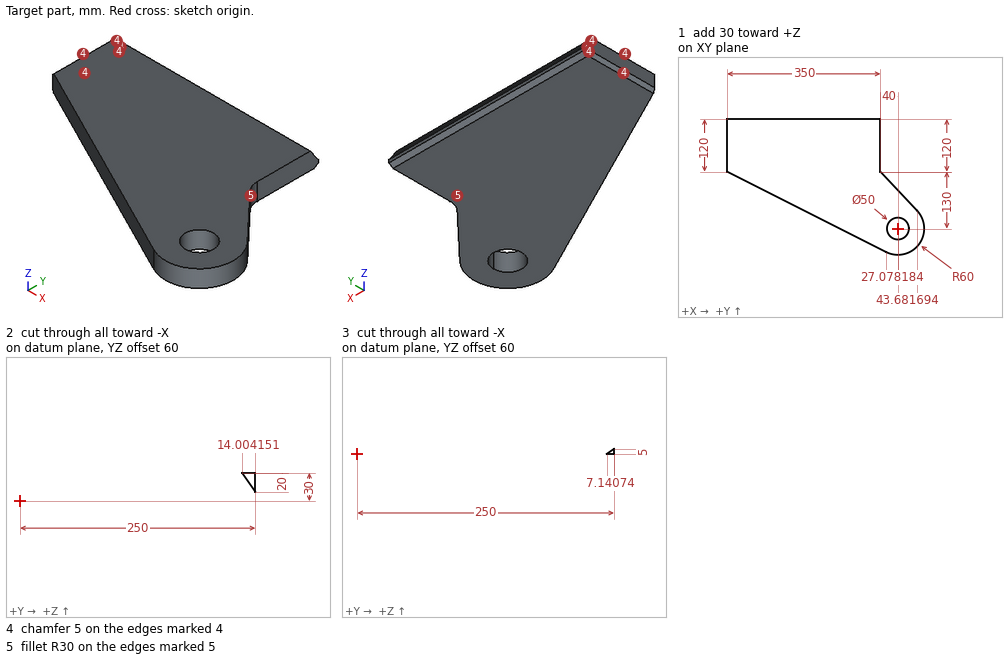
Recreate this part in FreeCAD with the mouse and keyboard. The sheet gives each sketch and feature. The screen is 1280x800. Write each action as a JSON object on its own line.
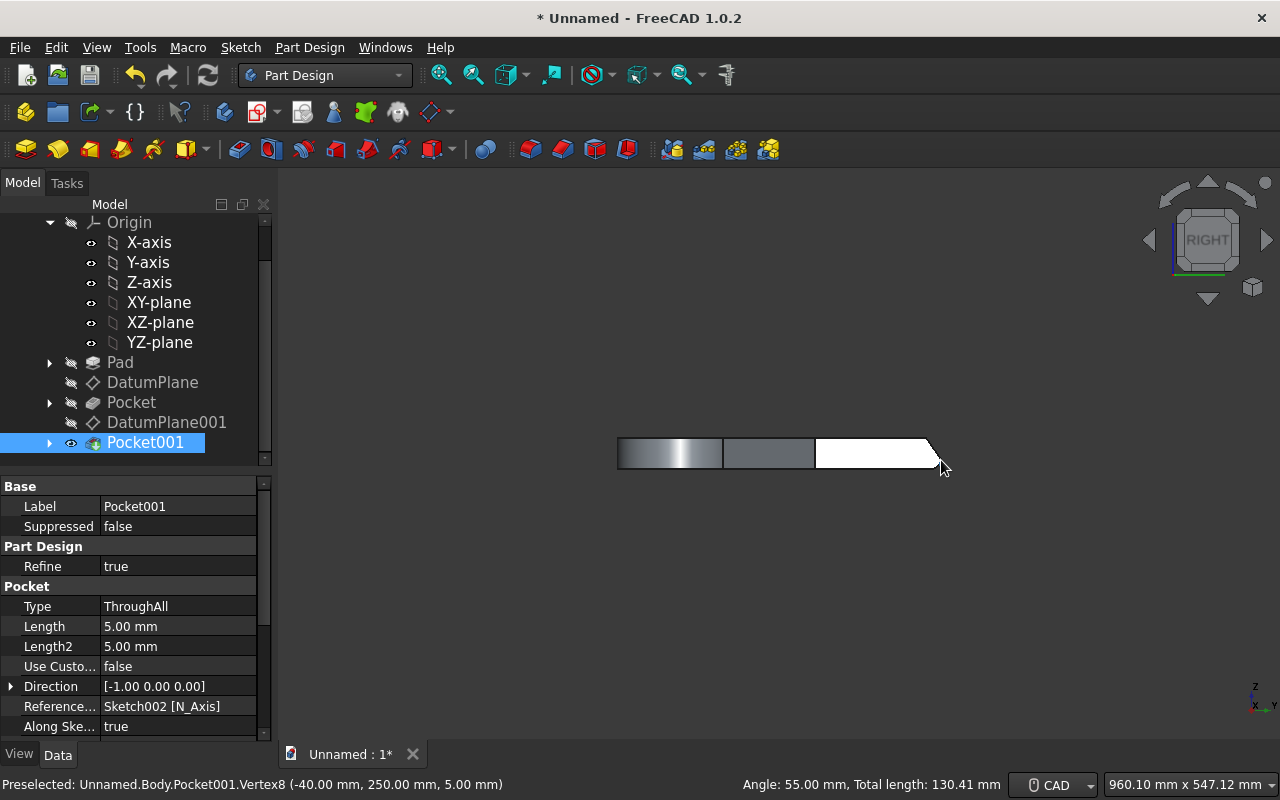
{"action": "key", "text": "5"}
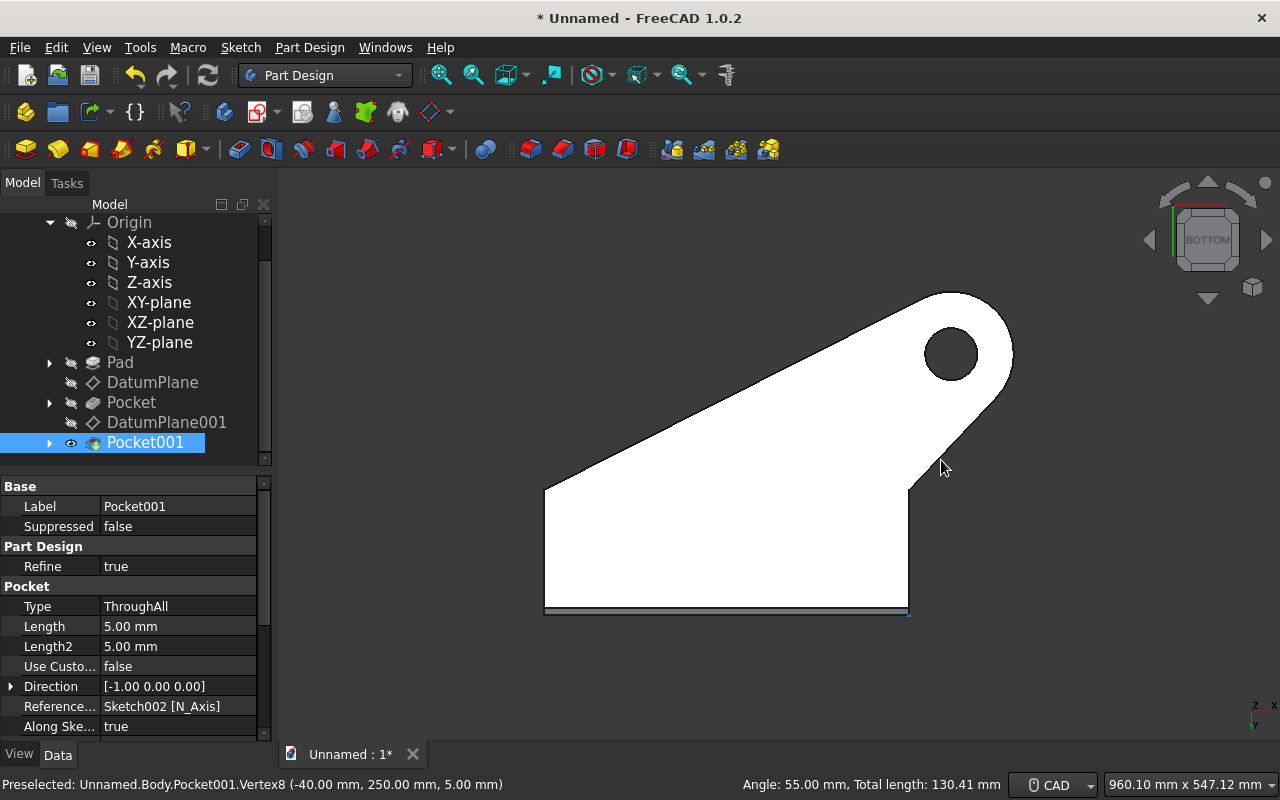
{"action": "left_click", "coordinate": [544, 548], "text": "ctrl"}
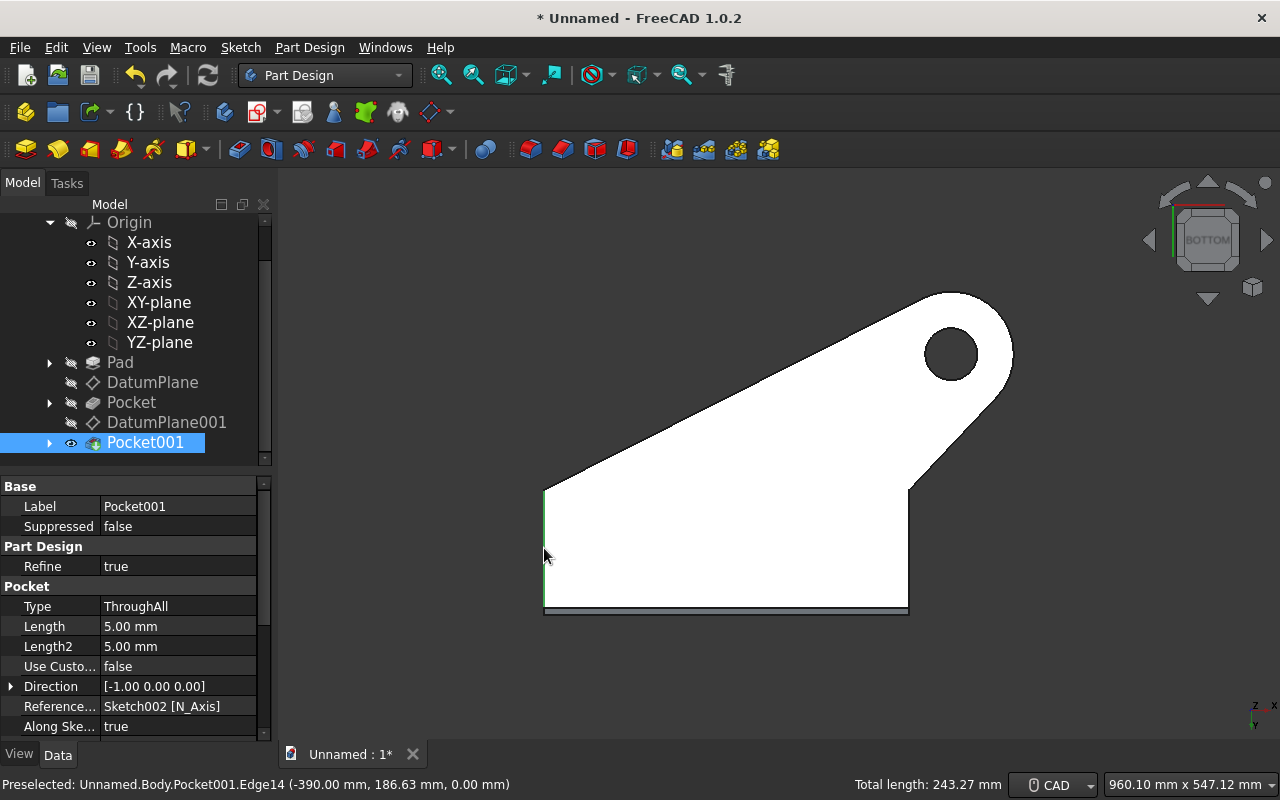
{"action": "left_click", "coordinate": [544, 613], "text": "ctrl"}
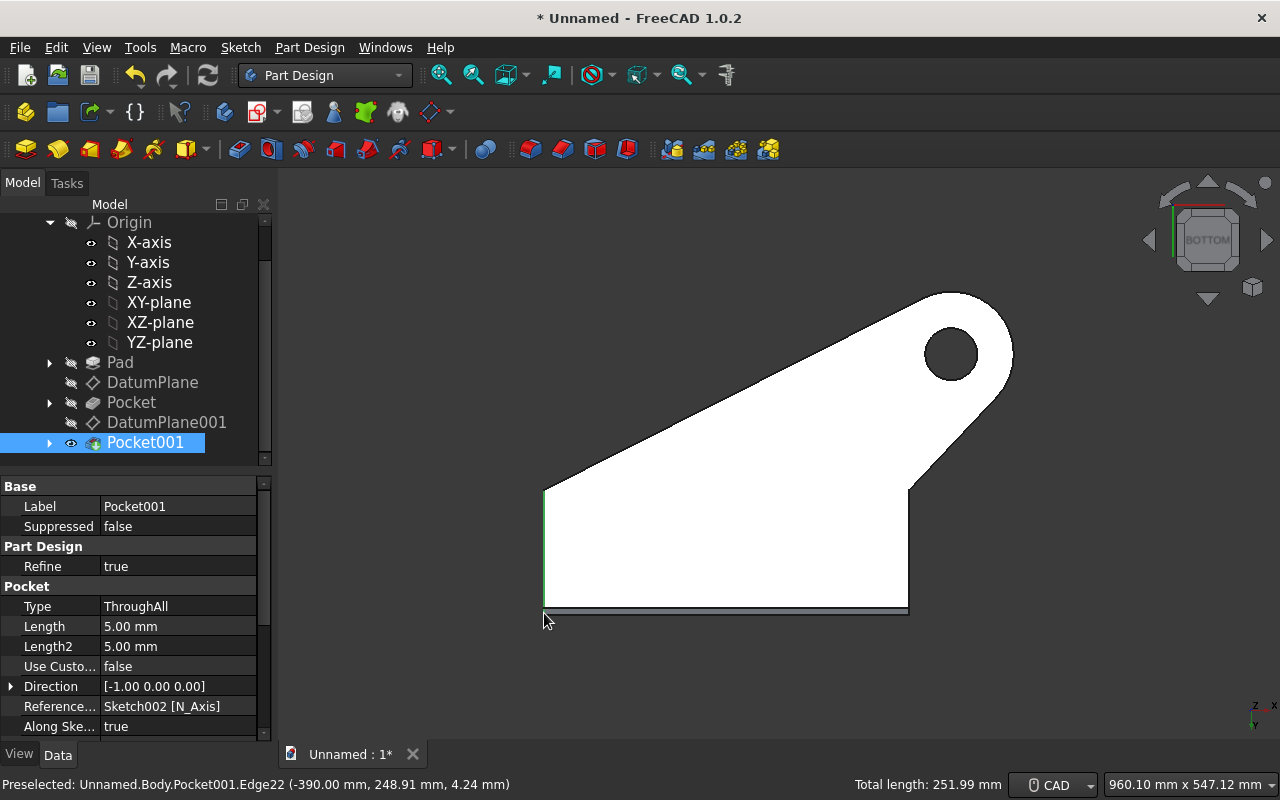
{"action": "scroll", "coordinate": [544, 614], "scroll_direction": "up", "scroll_amount": 11}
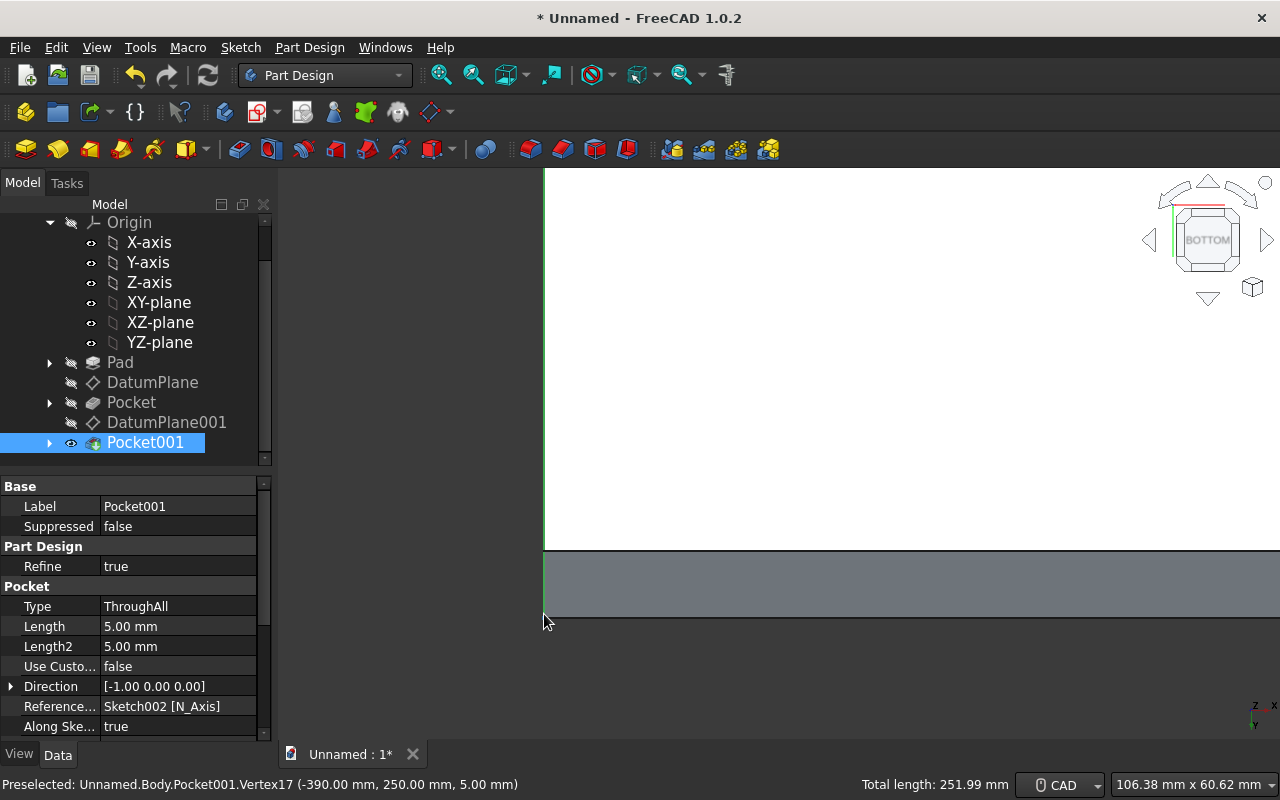
{"action": "left_click", "coordinate": [442, 76]}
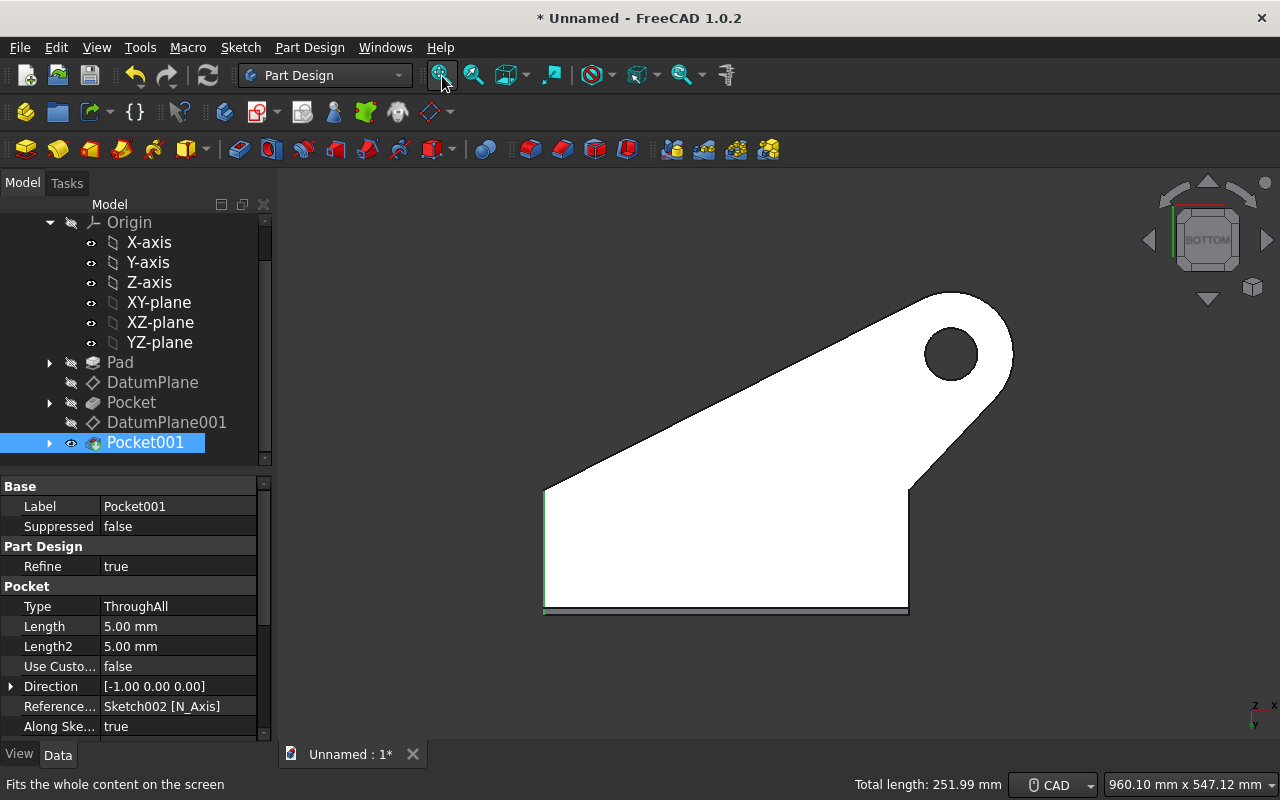
{"action": "key", "text": "4"}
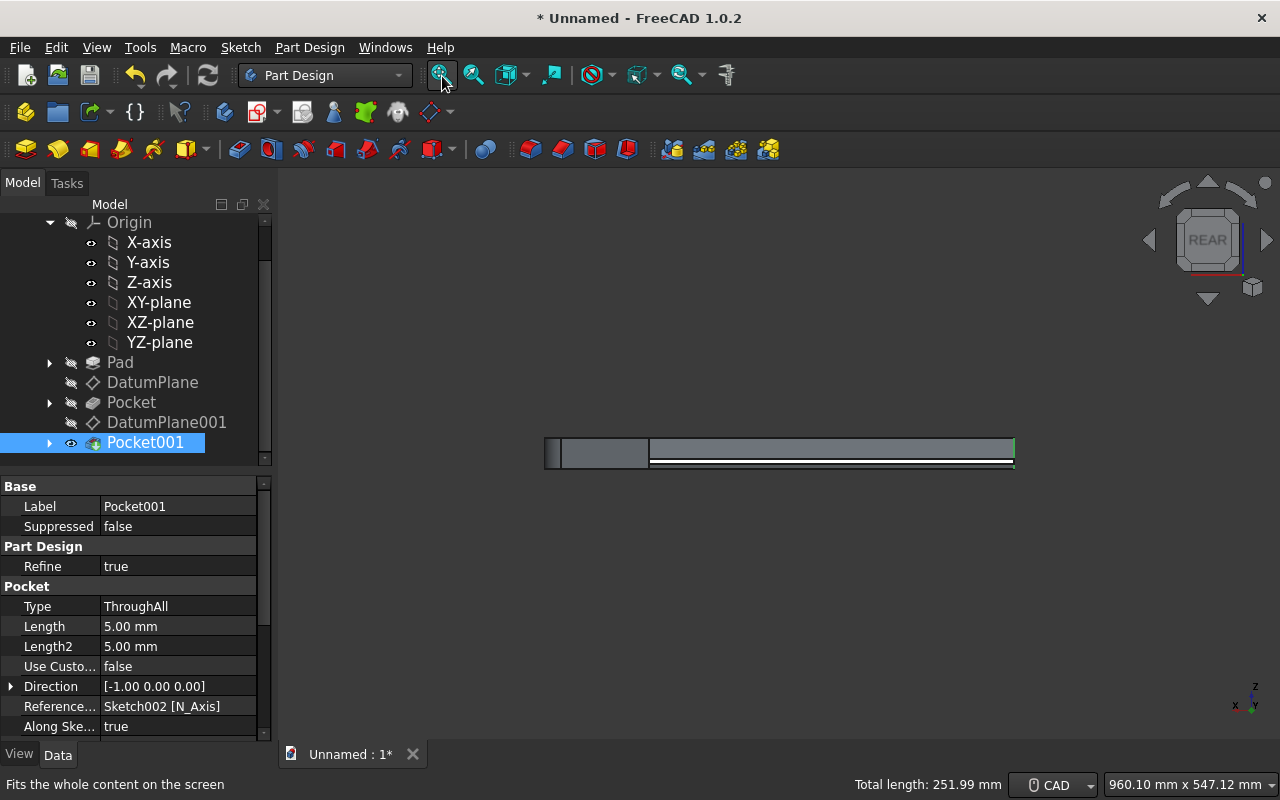
{"action": "scroll", "coordinate": [1014, 460], "scroll_direction": "up", "scroll_amount": 11}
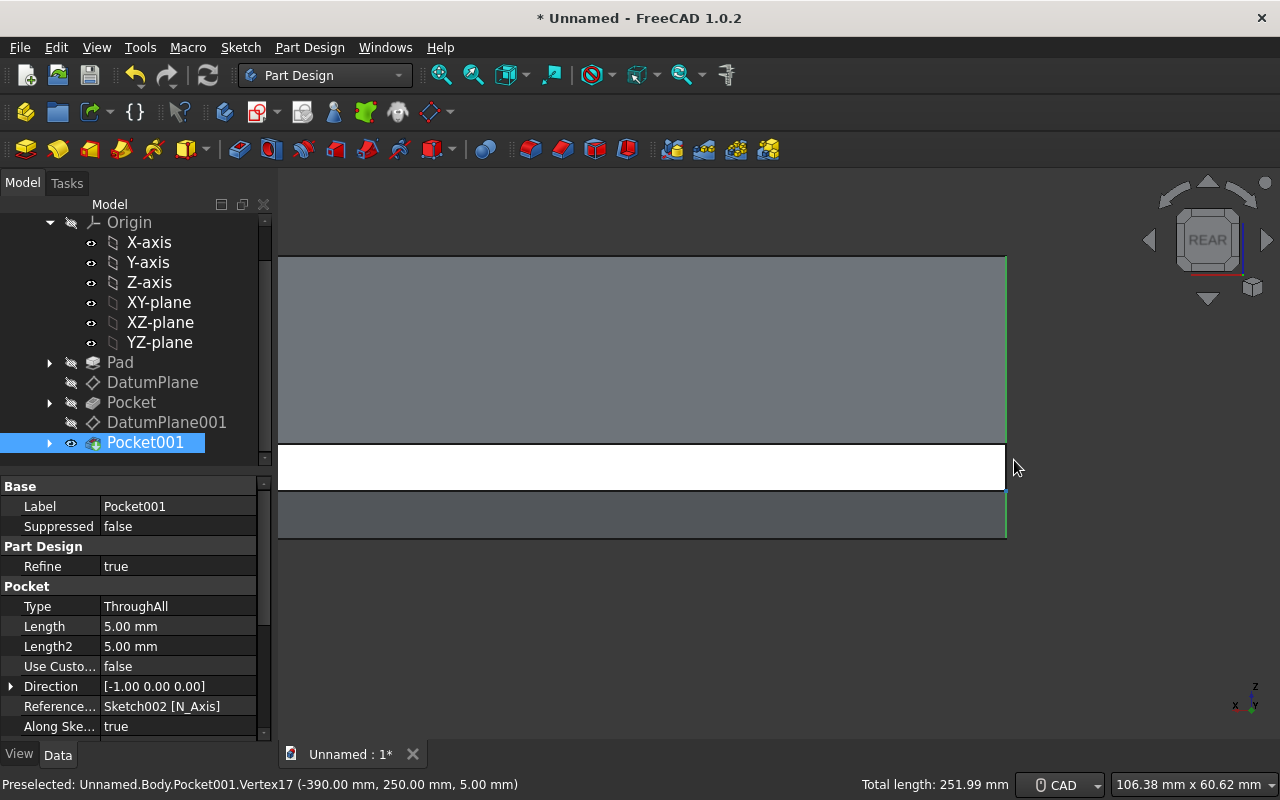
{"action": "left_click", "coordinate": [1006, 467], "text": "ctrl"}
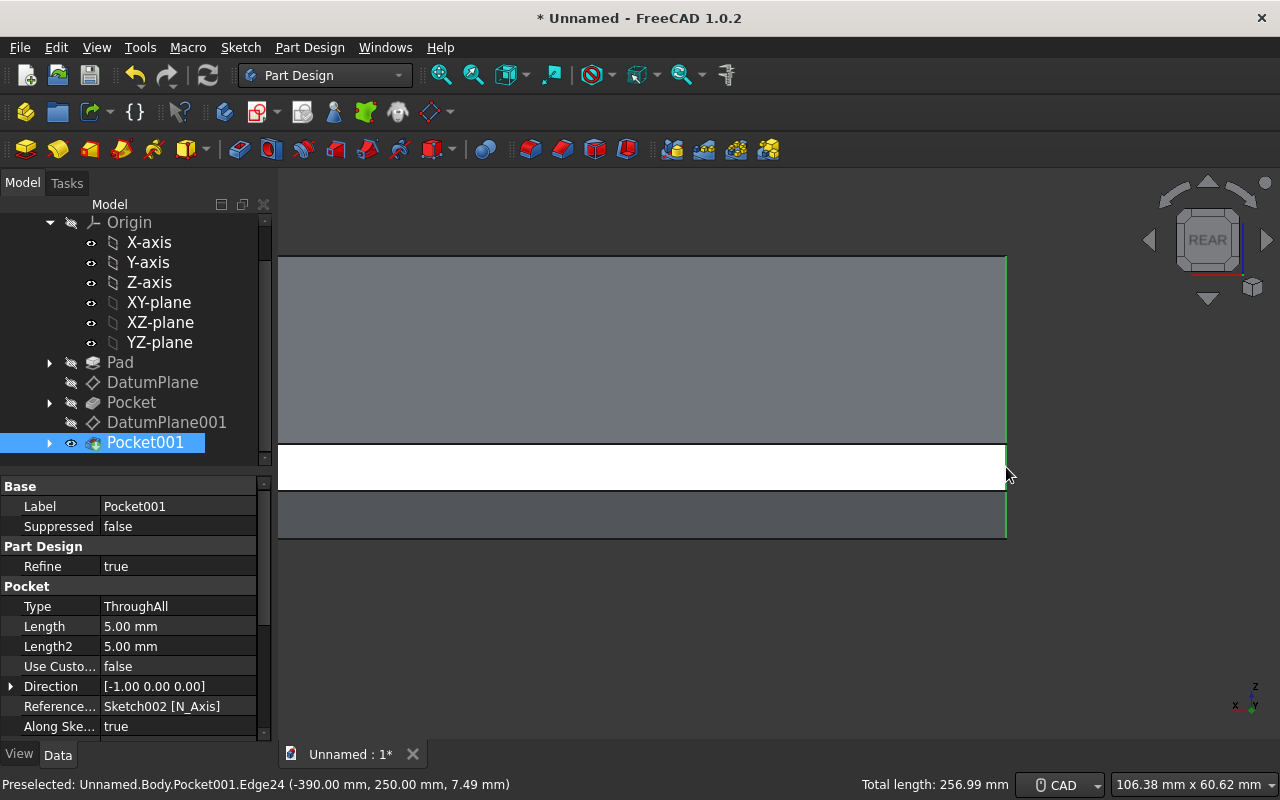
{"action": "left_click", "coordinate": [564, 150]}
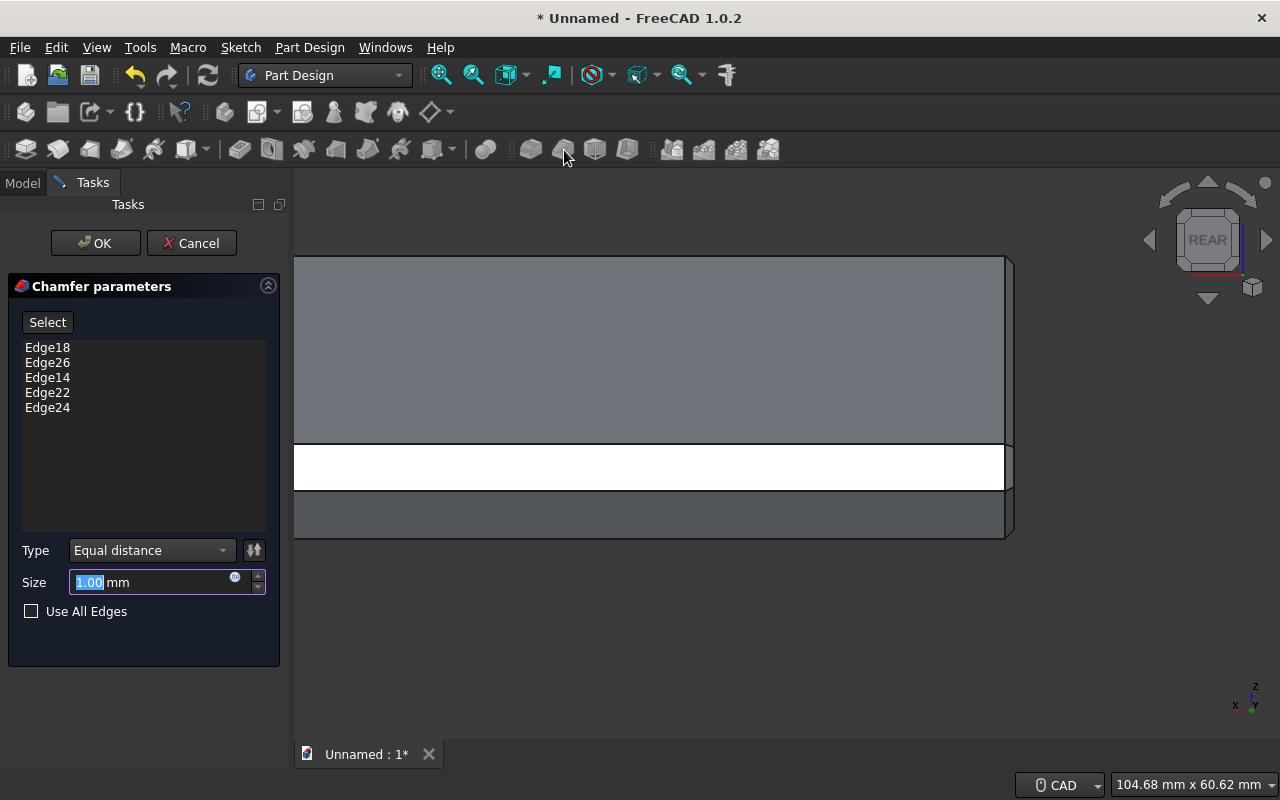
{"action": "type", "text": "5"}
{"action": "key", "text": "Tab"}